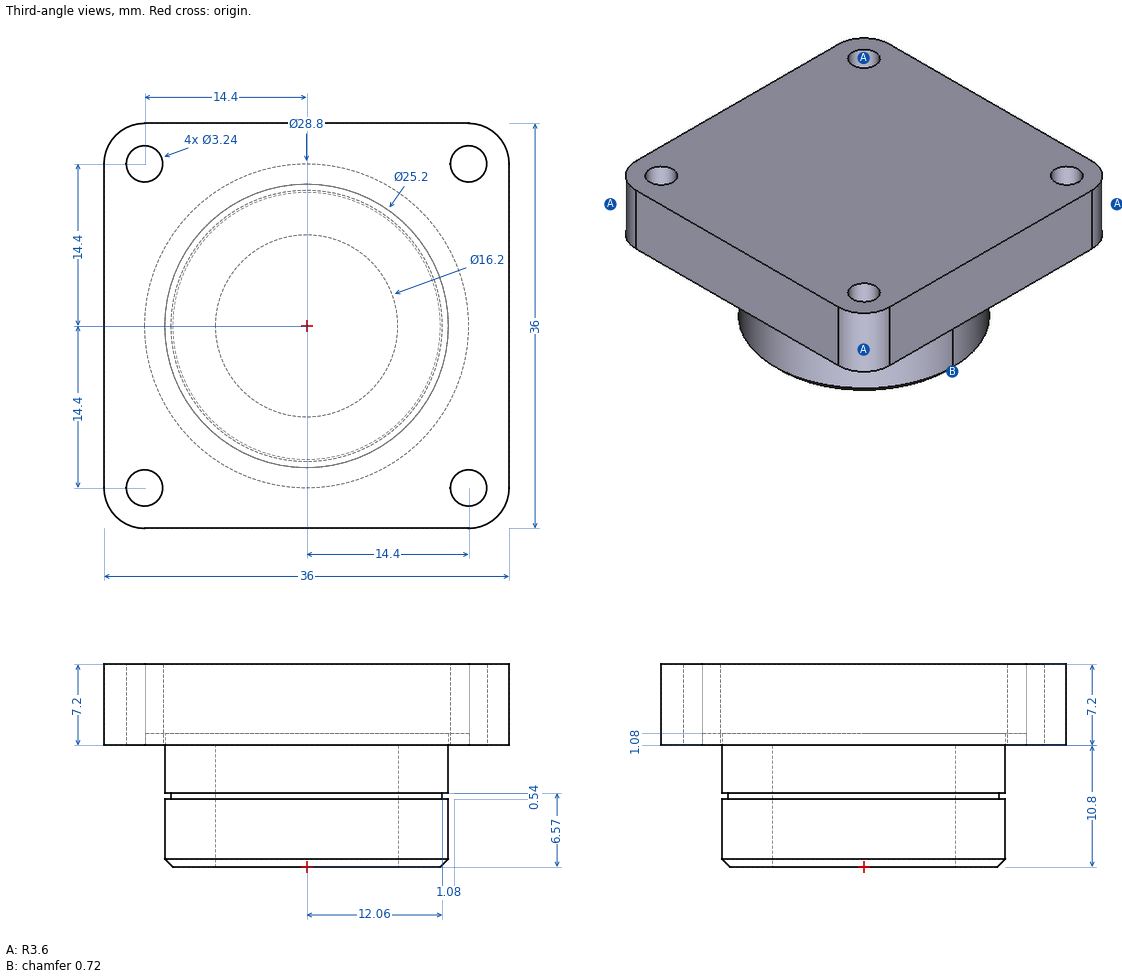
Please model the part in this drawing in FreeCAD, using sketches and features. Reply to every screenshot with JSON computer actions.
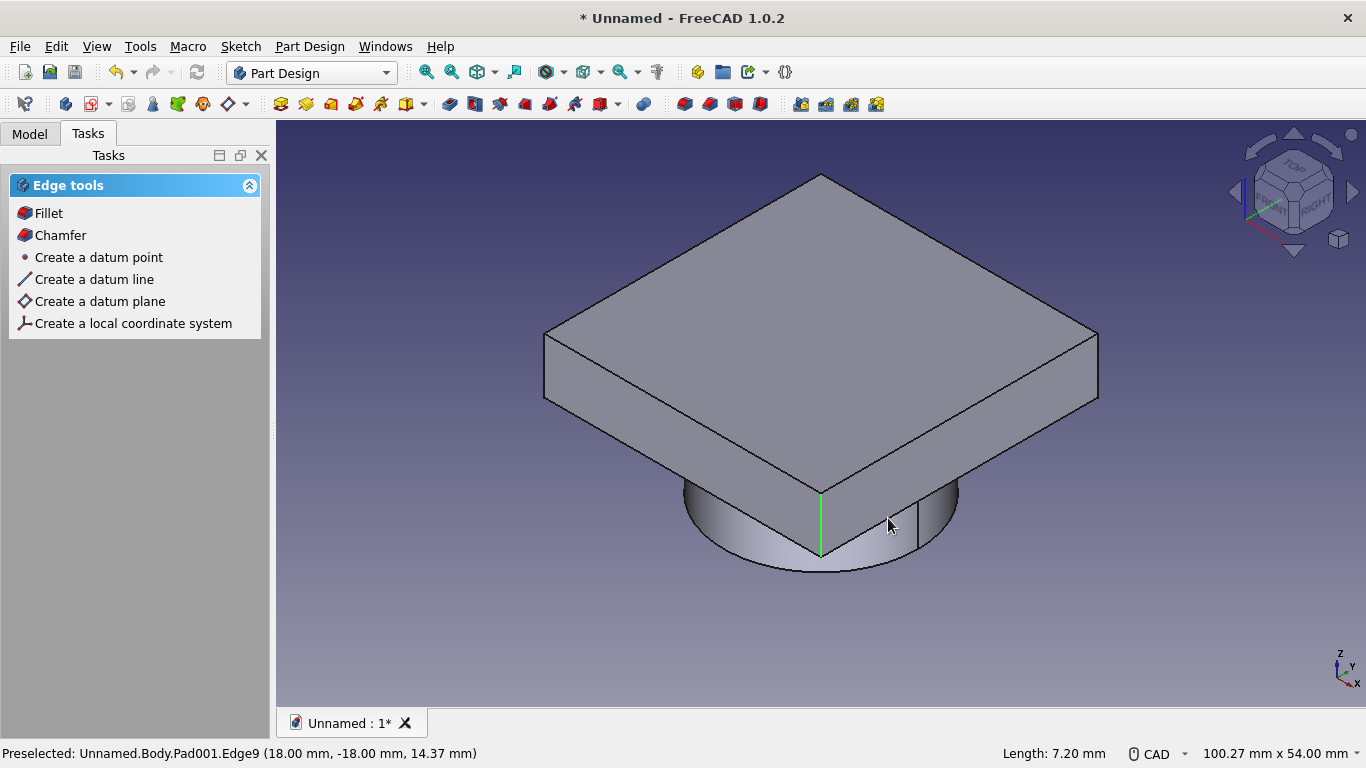
{"action": "key", "text": "2"}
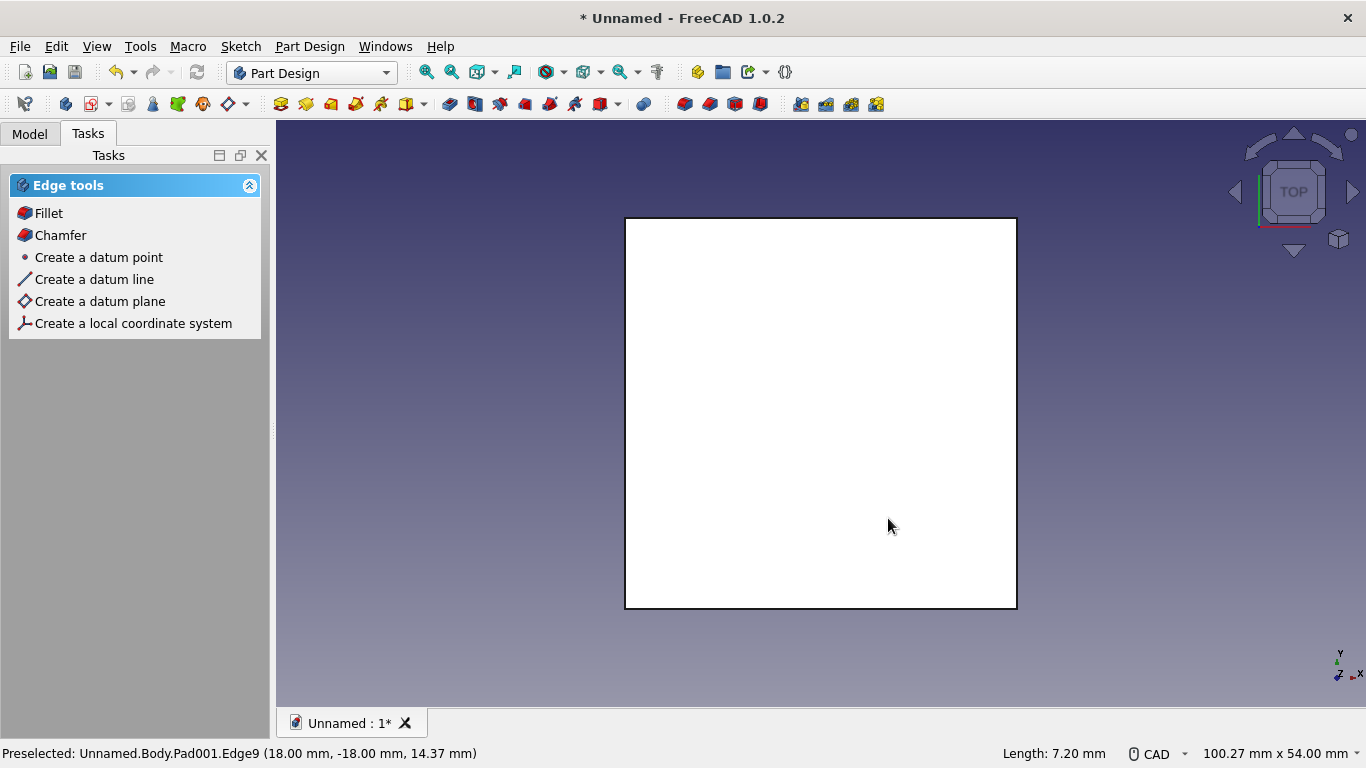
{"action": "key", "text": "1"}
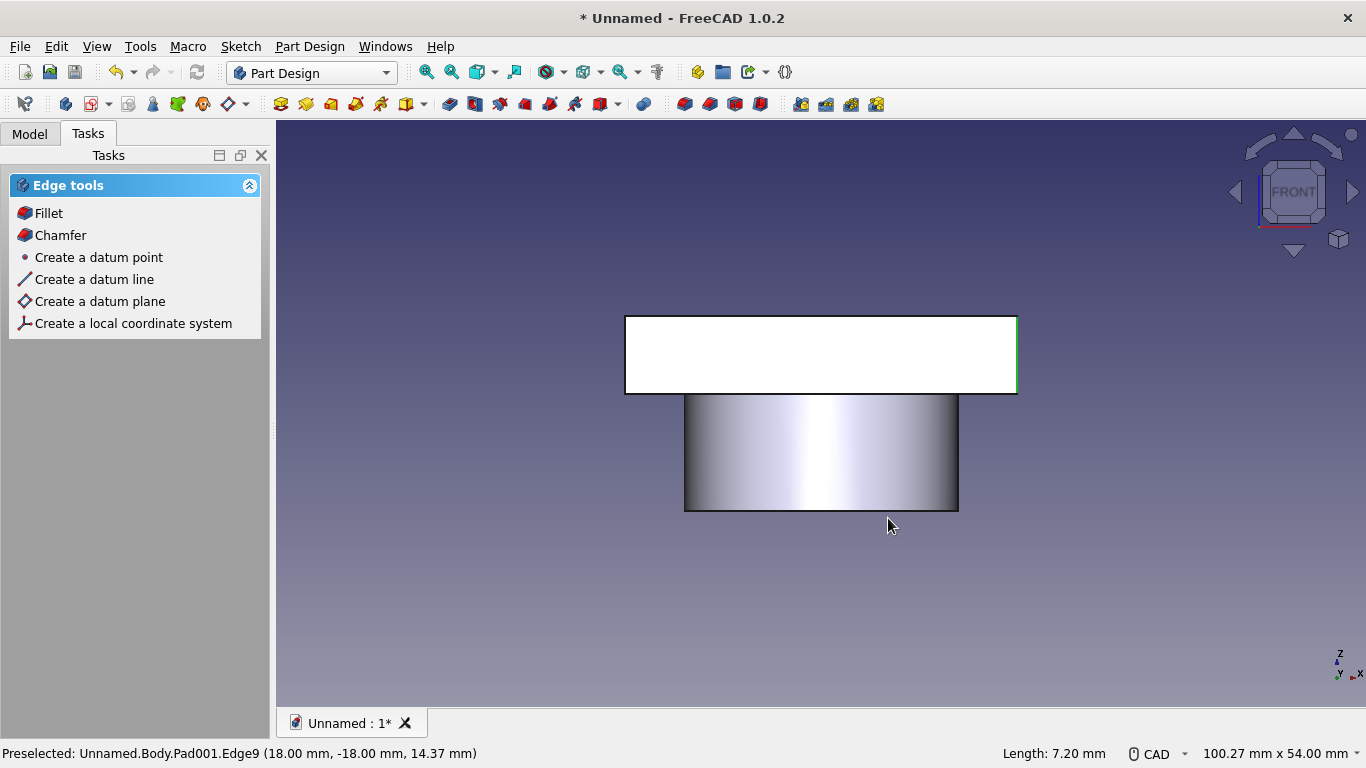
{"action": "left_click", "coordinate": [427, 72]}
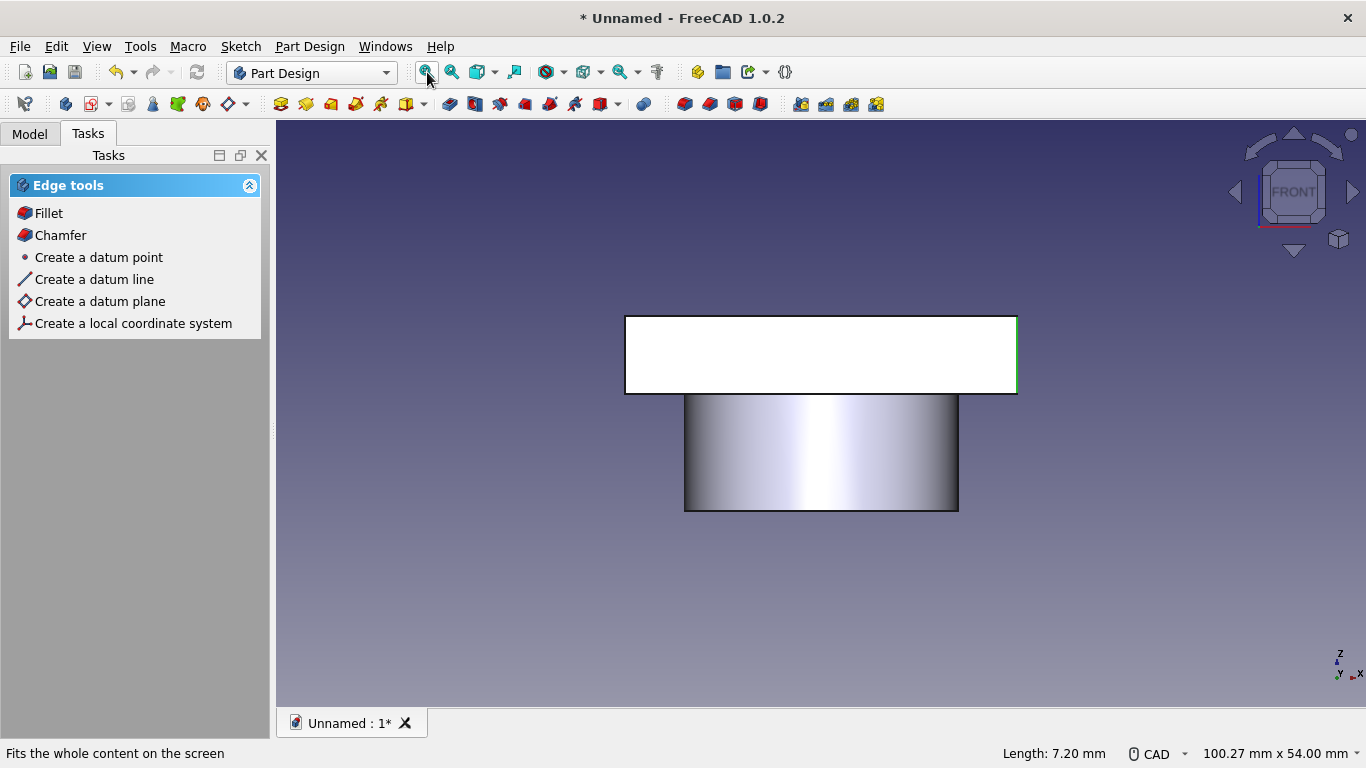
{"action": "left_click", "coordinate": [625, 354], "text": "ctrl"}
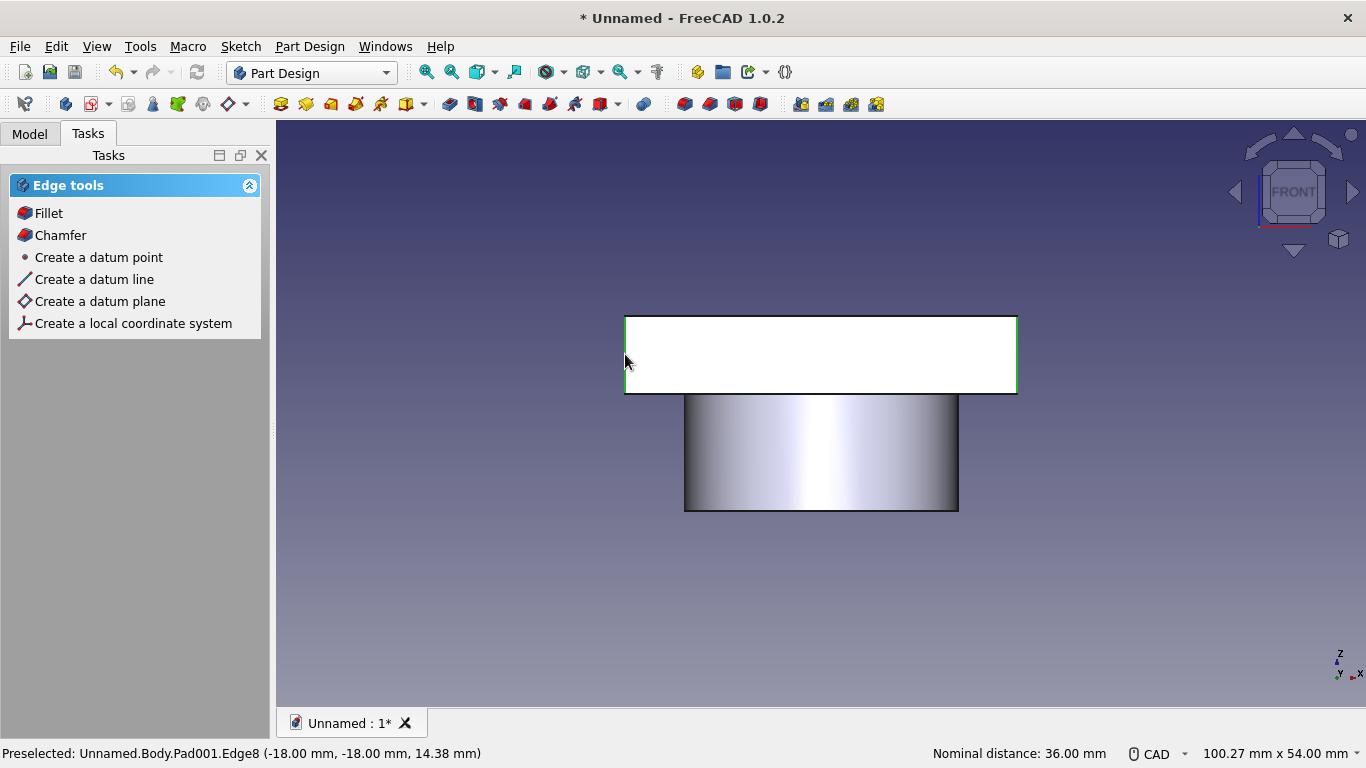
{"action": "key", "text": "3"}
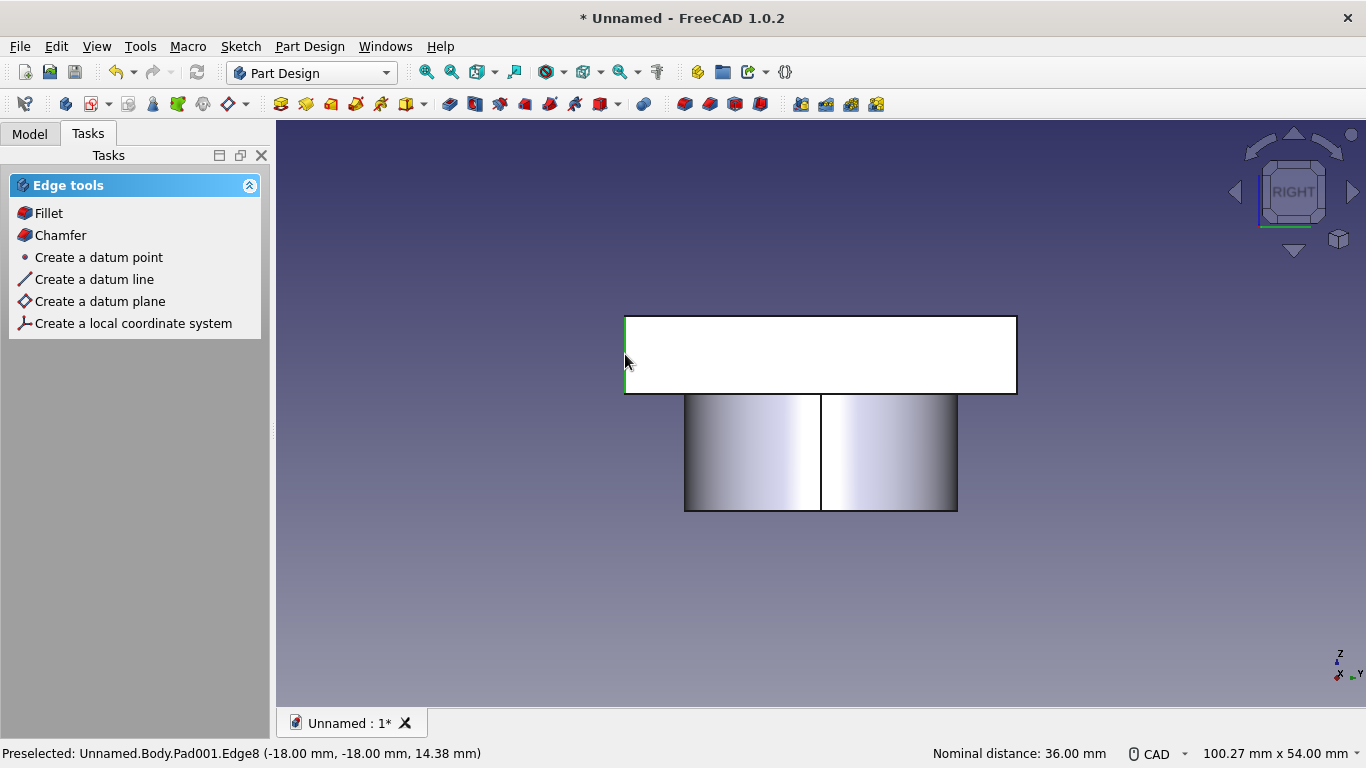
{"action": "left_click", "coordinate": [427, 72]}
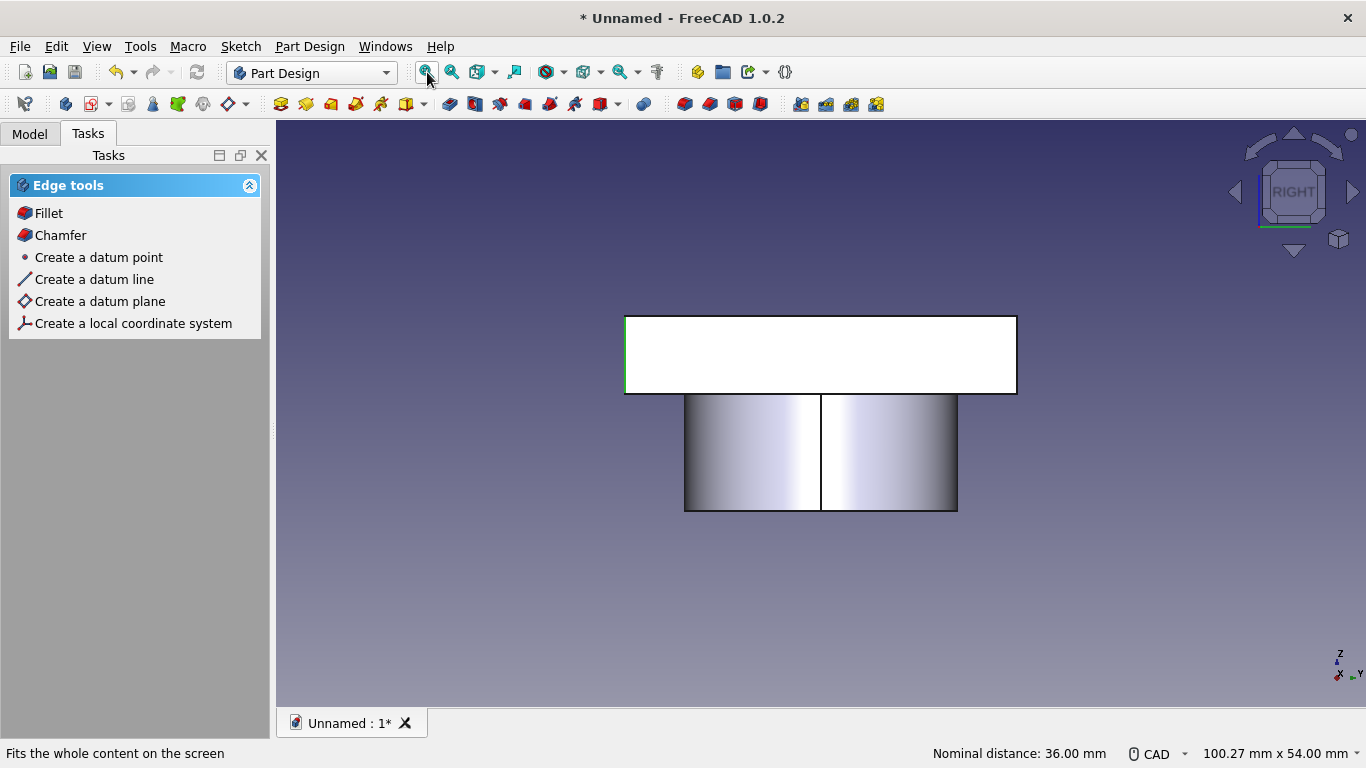
{"action": "left_click", "coordinate": [1017, 354], "text": "ctrl"}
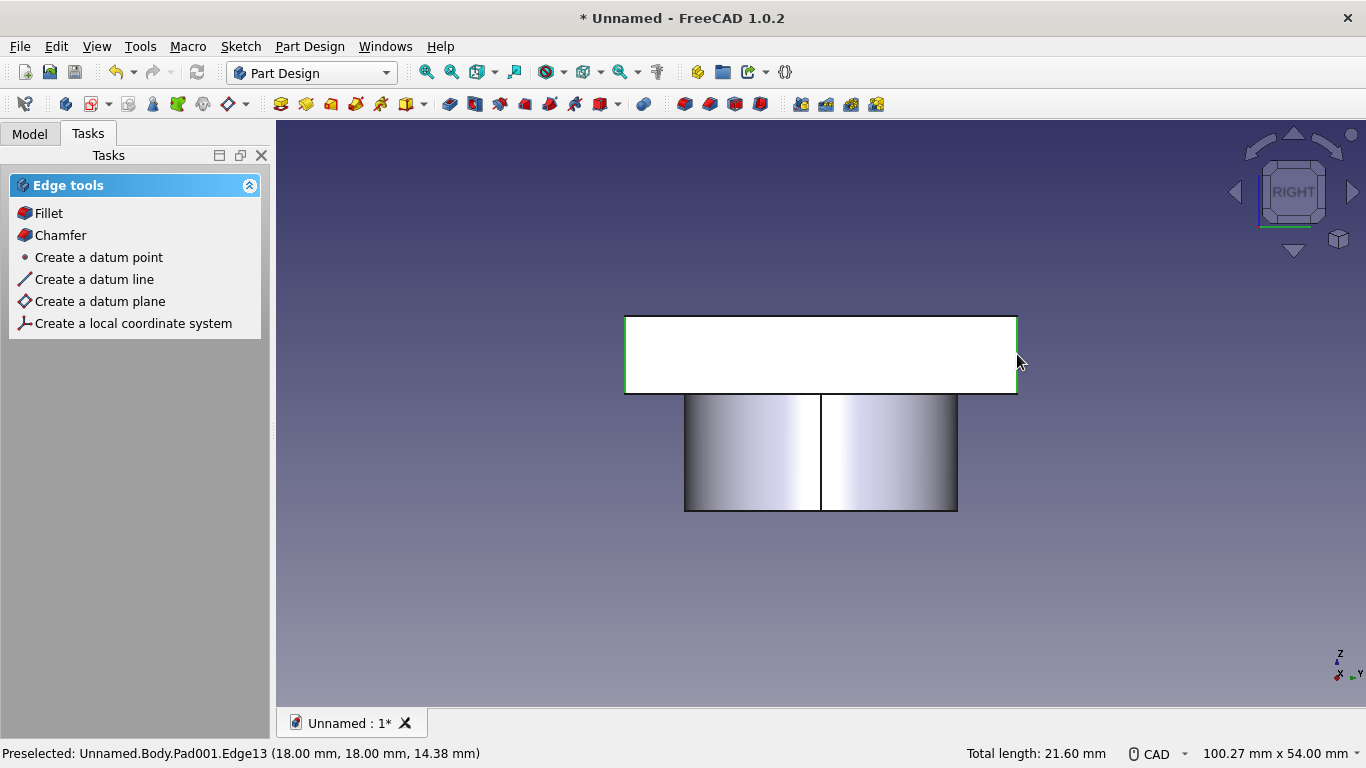
{"action": "key", "text": "5"}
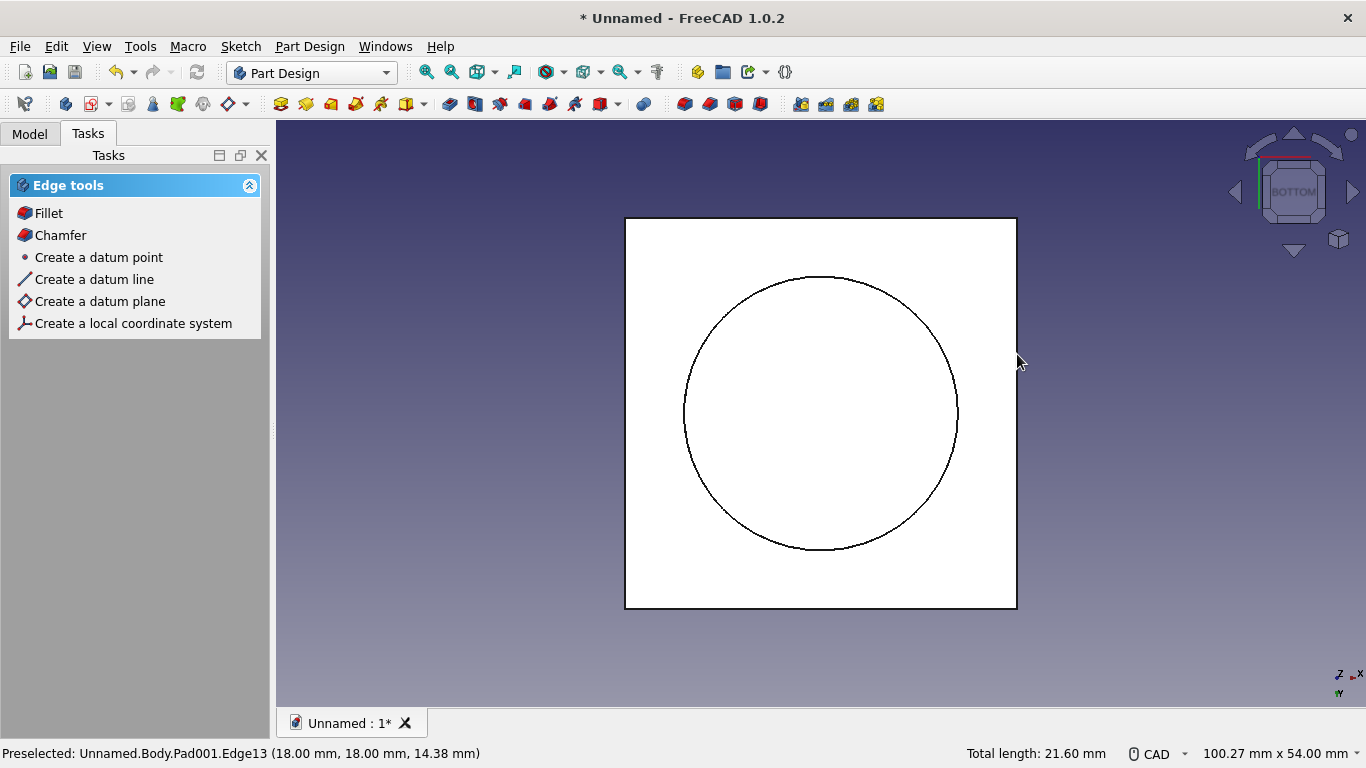
{"action": "key", "text": "4"}